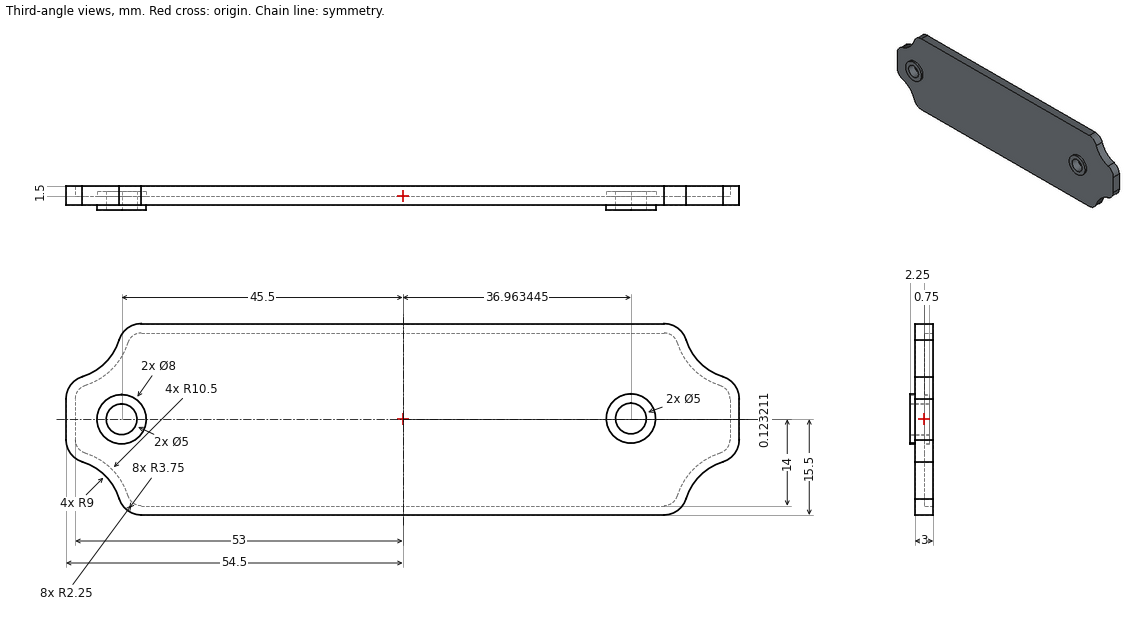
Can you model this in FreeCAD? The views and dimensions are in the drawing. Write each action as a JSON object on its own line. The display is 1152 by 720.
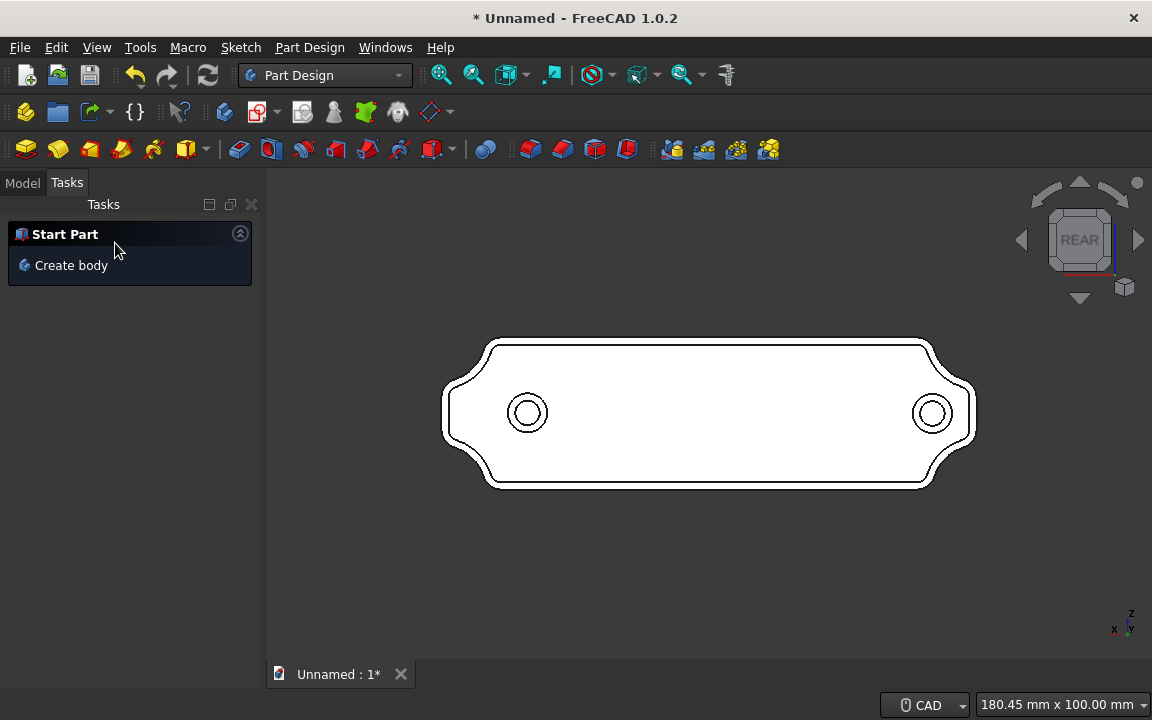
{"action": "left_click", "coordinate": [258, 112]}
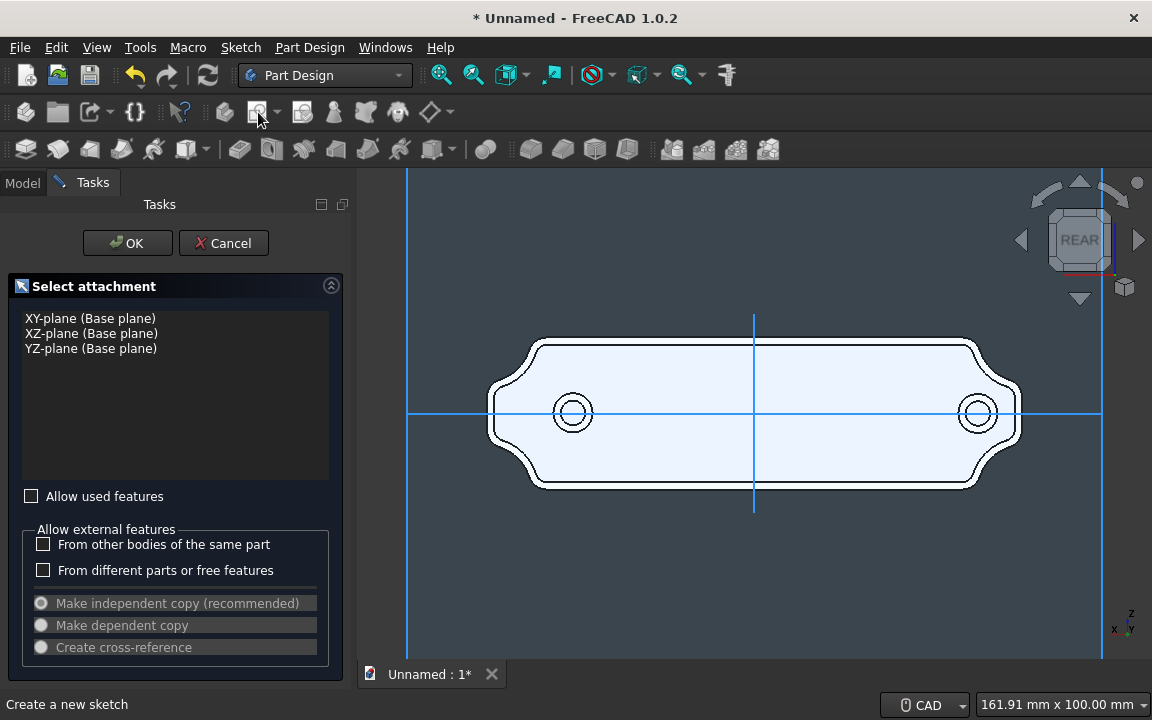
{"action": "left_click", "coordinate": [82, 334]}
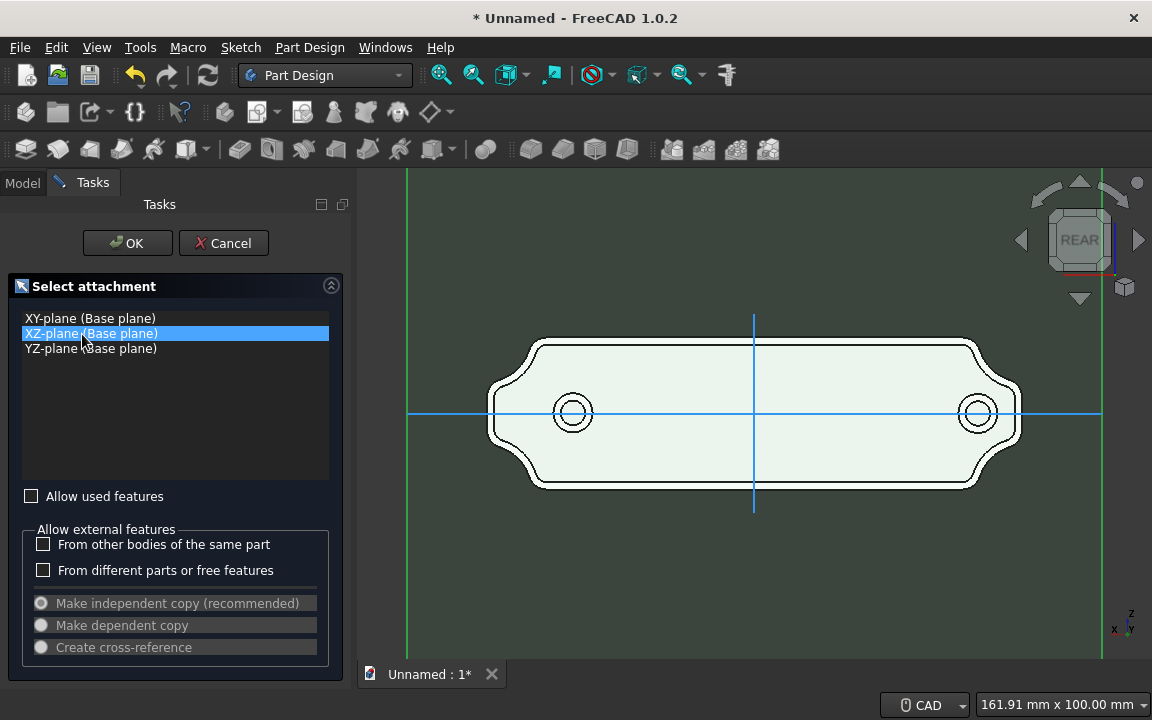
{"action": "left_click", "coordinate": [128, 243]}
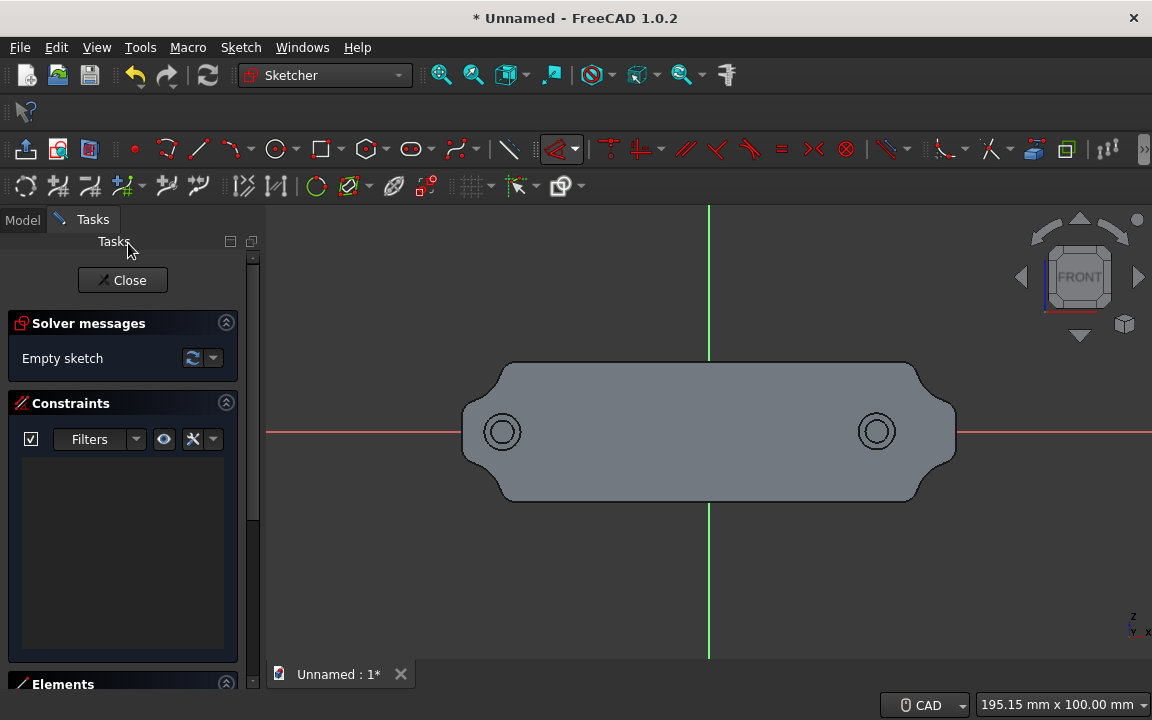
{"action": "left_click", "coordinate": [90, 150]}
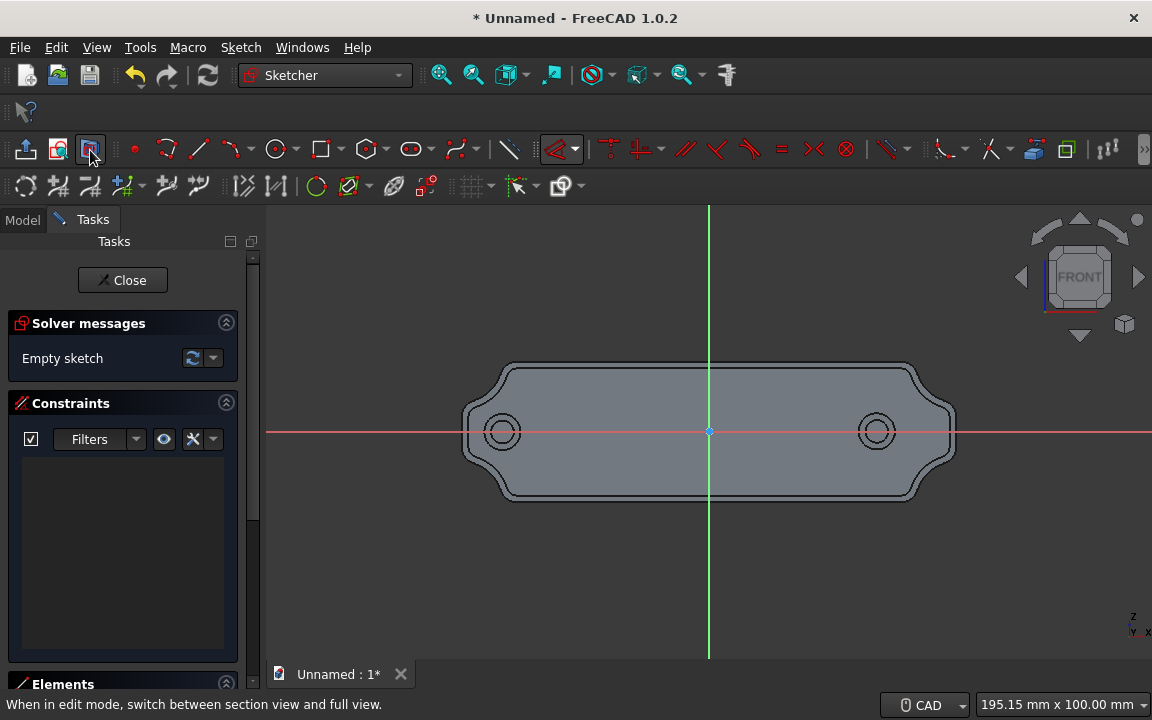
{"action": "left_click", "coordinate": [276, 150]}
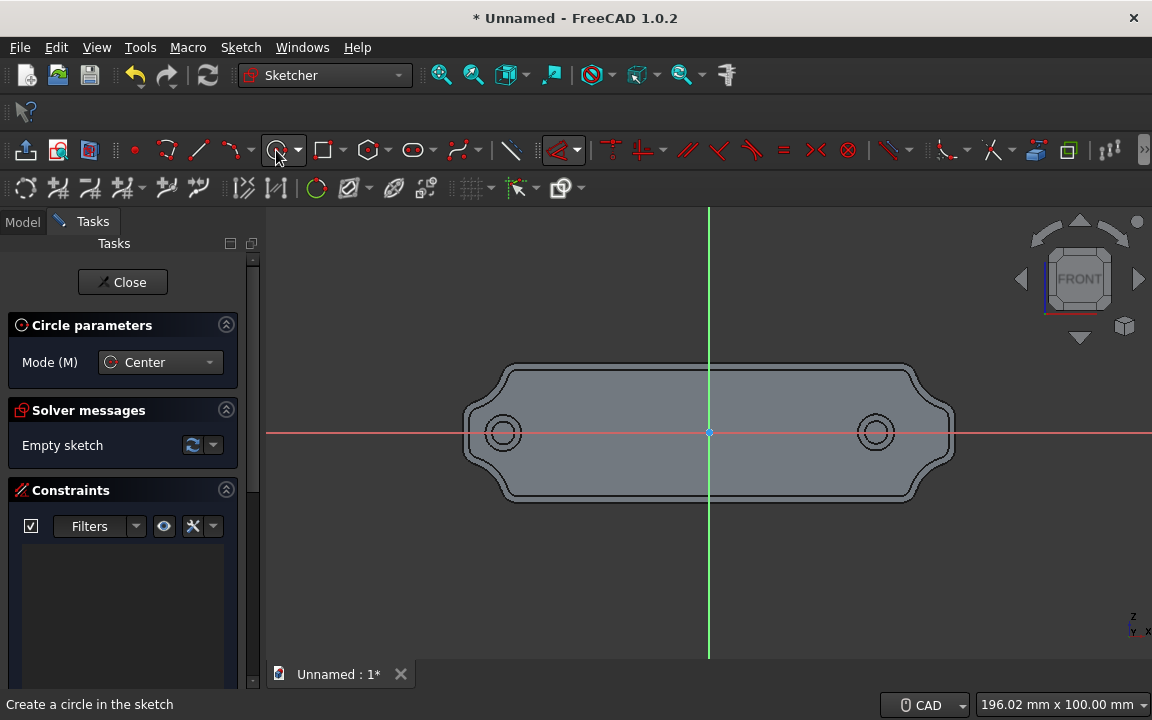
{"action": "scroll", "coordinate": [876, 432], "scroll_direction": "up", "scroll_amount": 17}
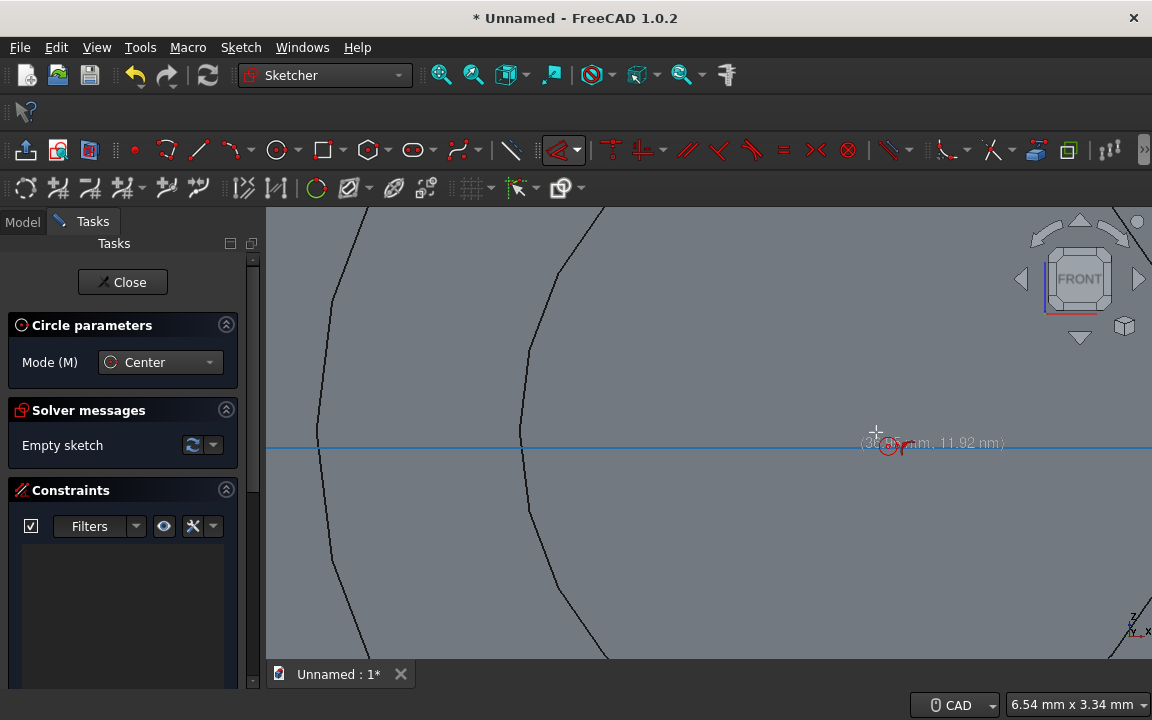
{"action": "left_click", "coordinate": [858, 431]}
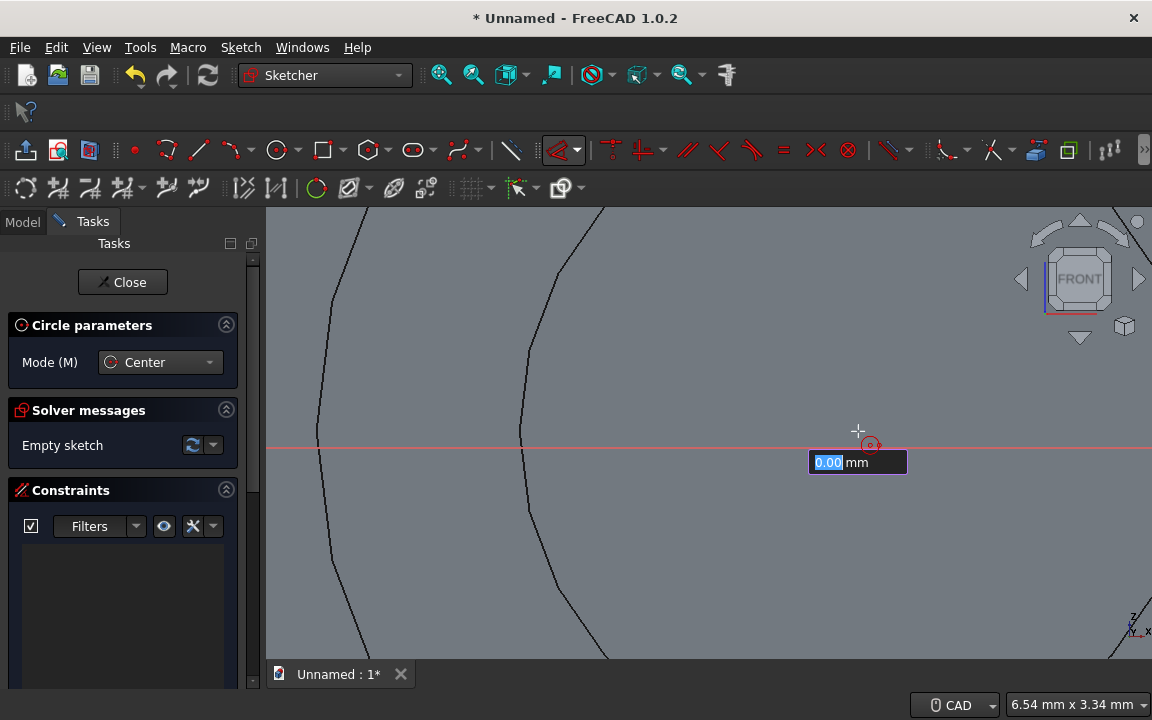
{"action": "scroll", "coordinate": [922, 433], "scroll_direction": "down", "scroll_amount": 15}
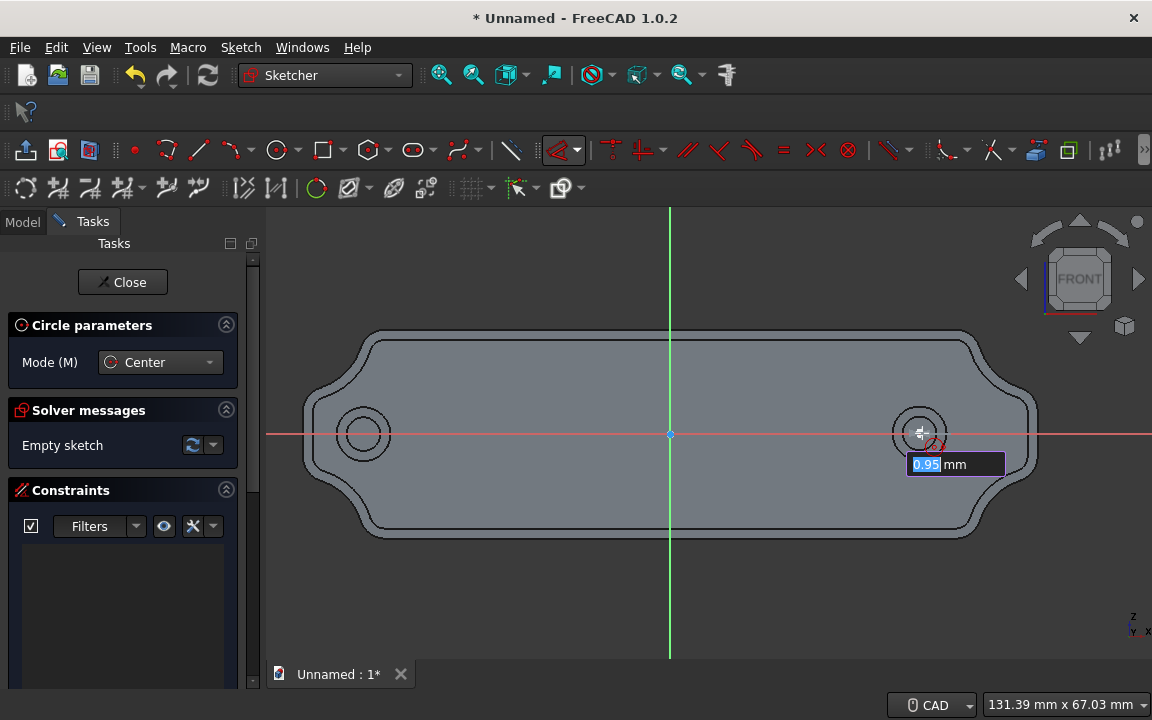
{"action": "scroll", "coordinate": [931, 421], "scroll_direction": "up", "scroll_amount": 2}
{"action": "mouse_move", "coordinate": [931, 421]}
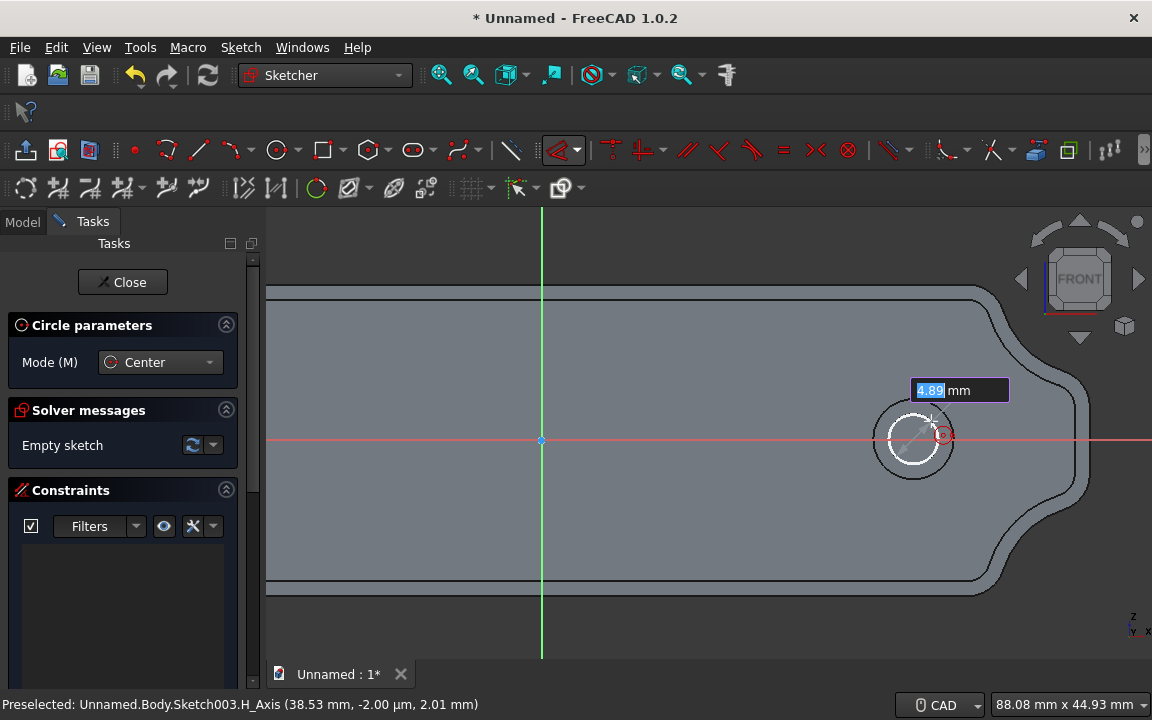
{"action": "type", "text": "5"}
{"action": "key", "text": "Return"}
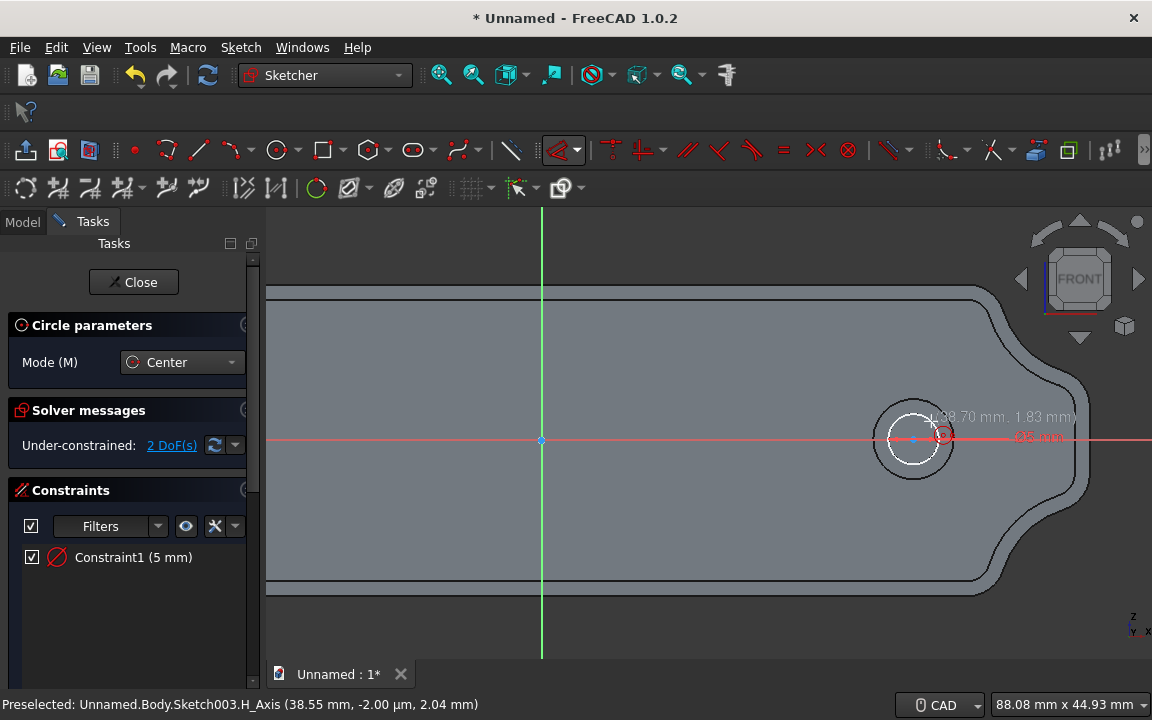
{"action": "scroll", "coordinate": [813, 425], "scroll_direction": "down", "scroll_amount": 3}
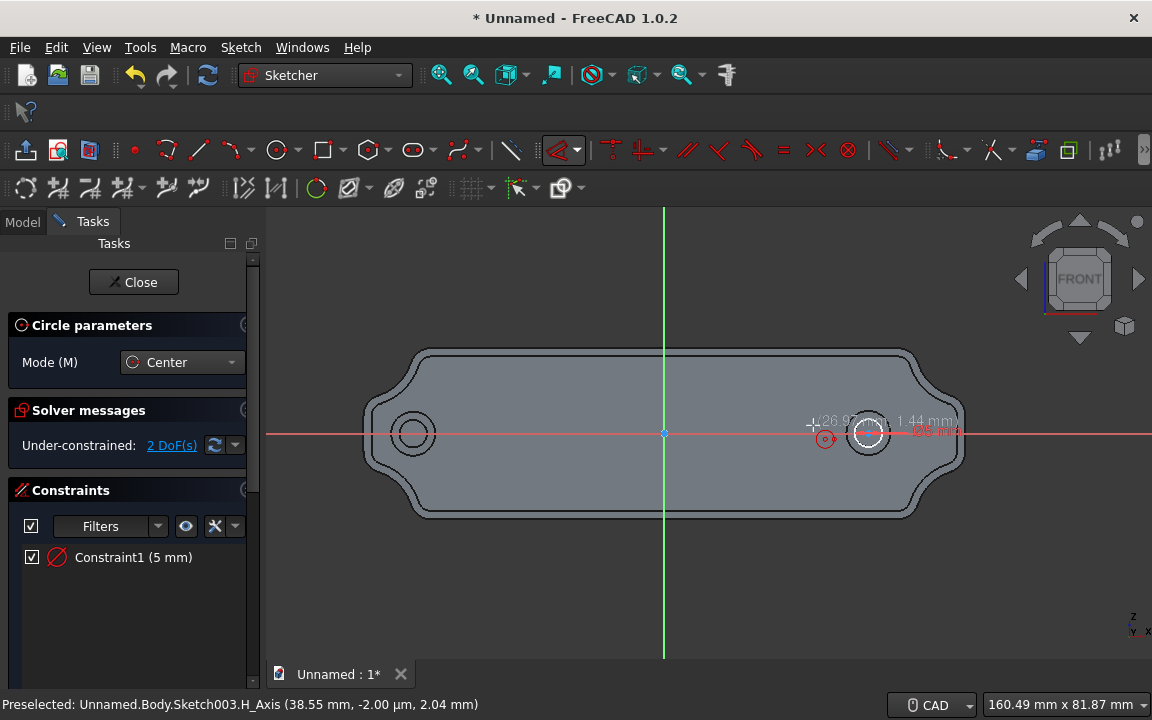
{"action": "scroll", "coordinate": [413, 434], "scroll_direction": "up", "scroll_amount": 3}